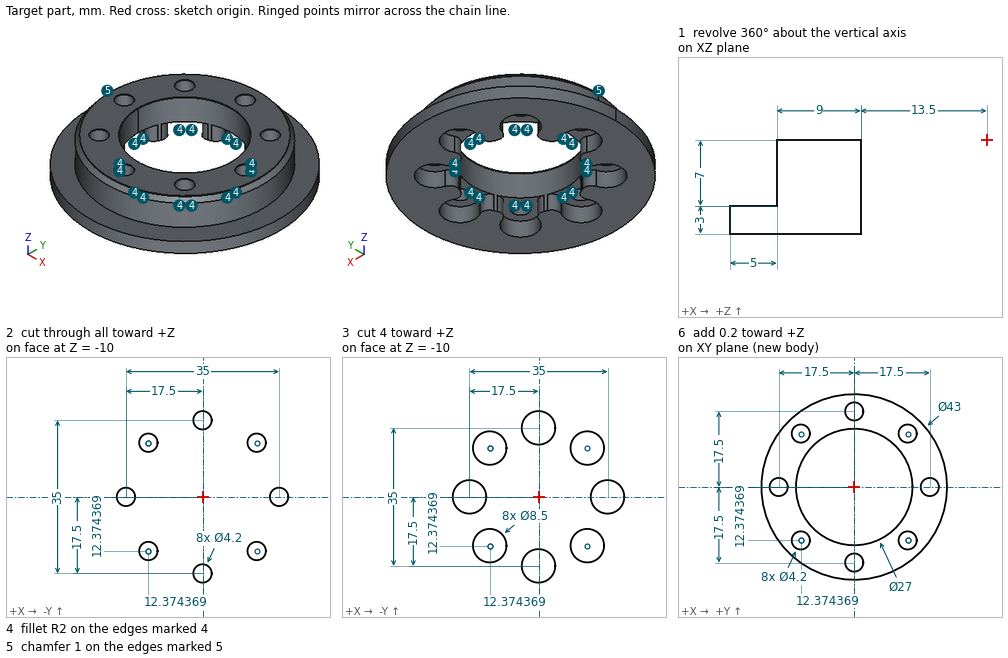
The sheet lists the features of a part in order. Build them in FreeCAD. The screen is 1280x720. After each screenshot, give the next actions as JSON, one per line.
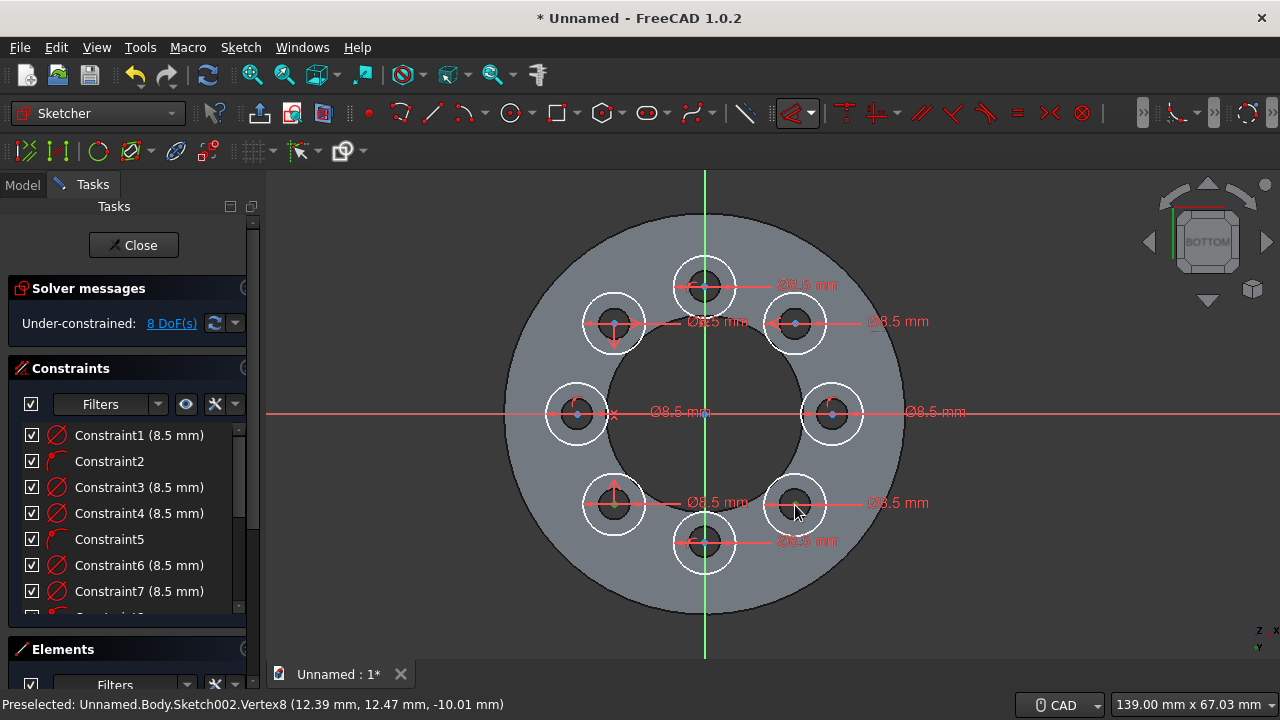
{"action": "left_click", "coordinate": [705, 476]}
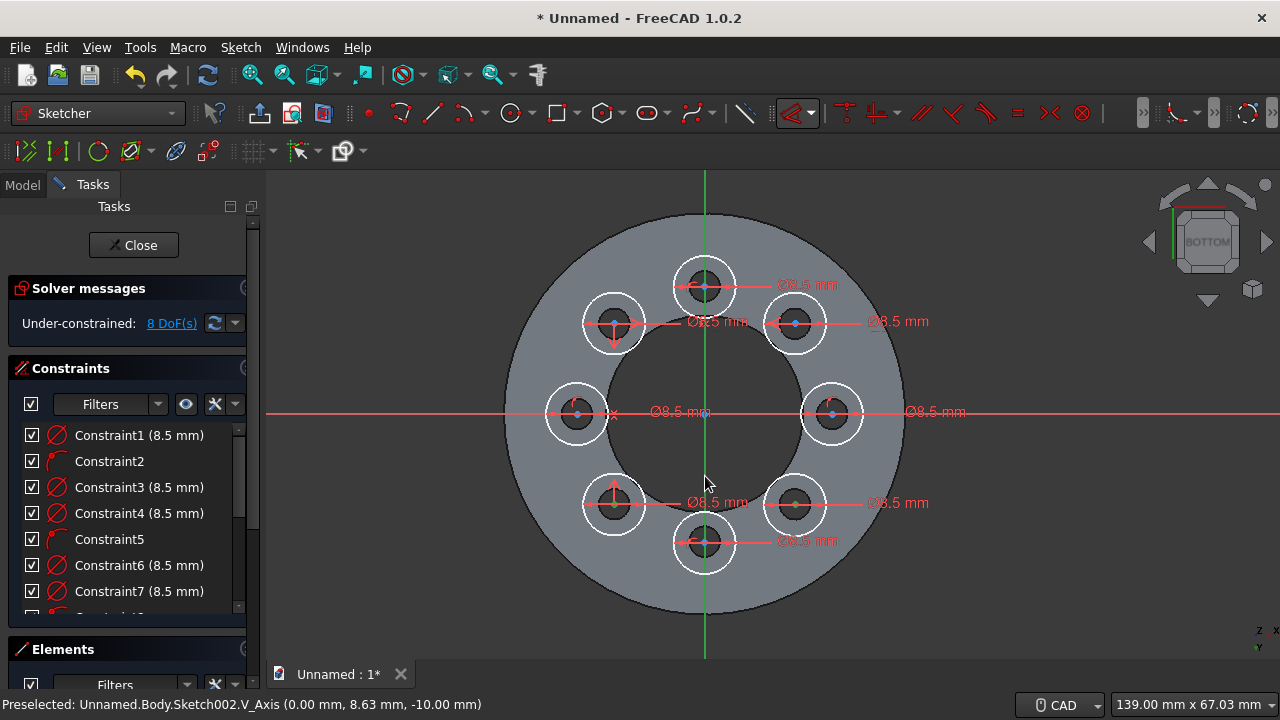
{"action": "key", "text": "s"}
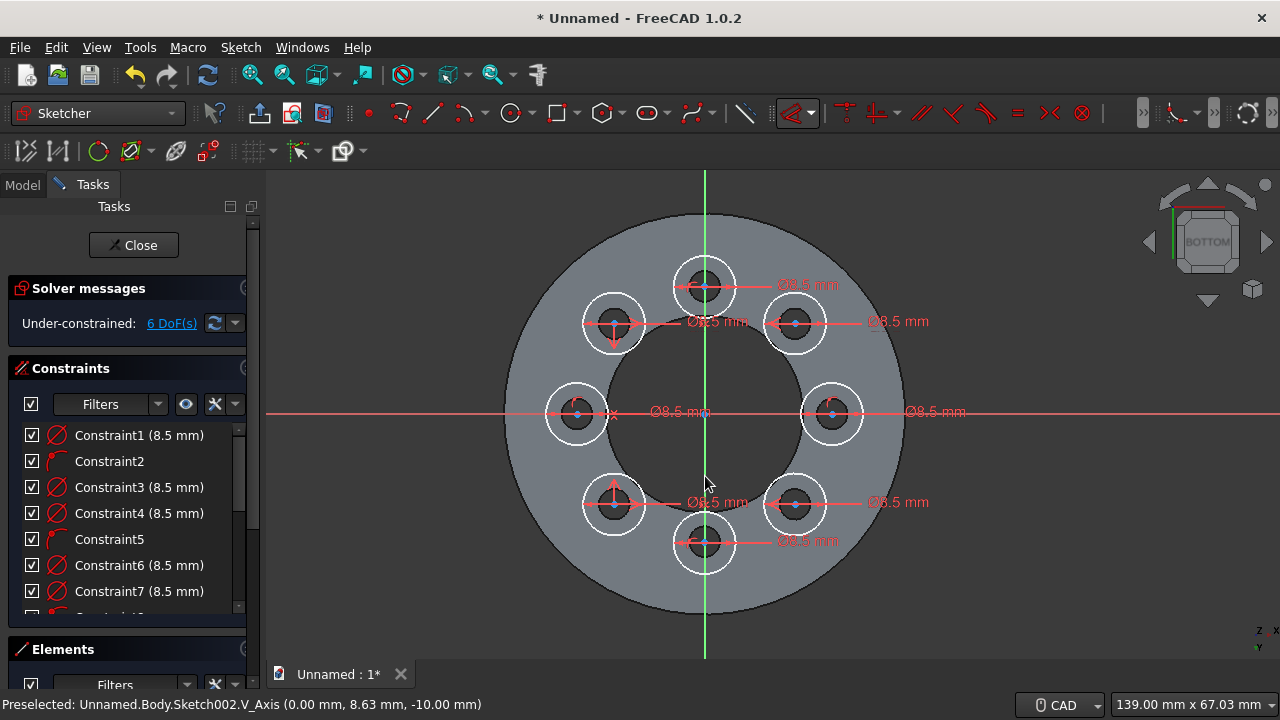
{"action": "left_click", "coordinate": [705, 543]}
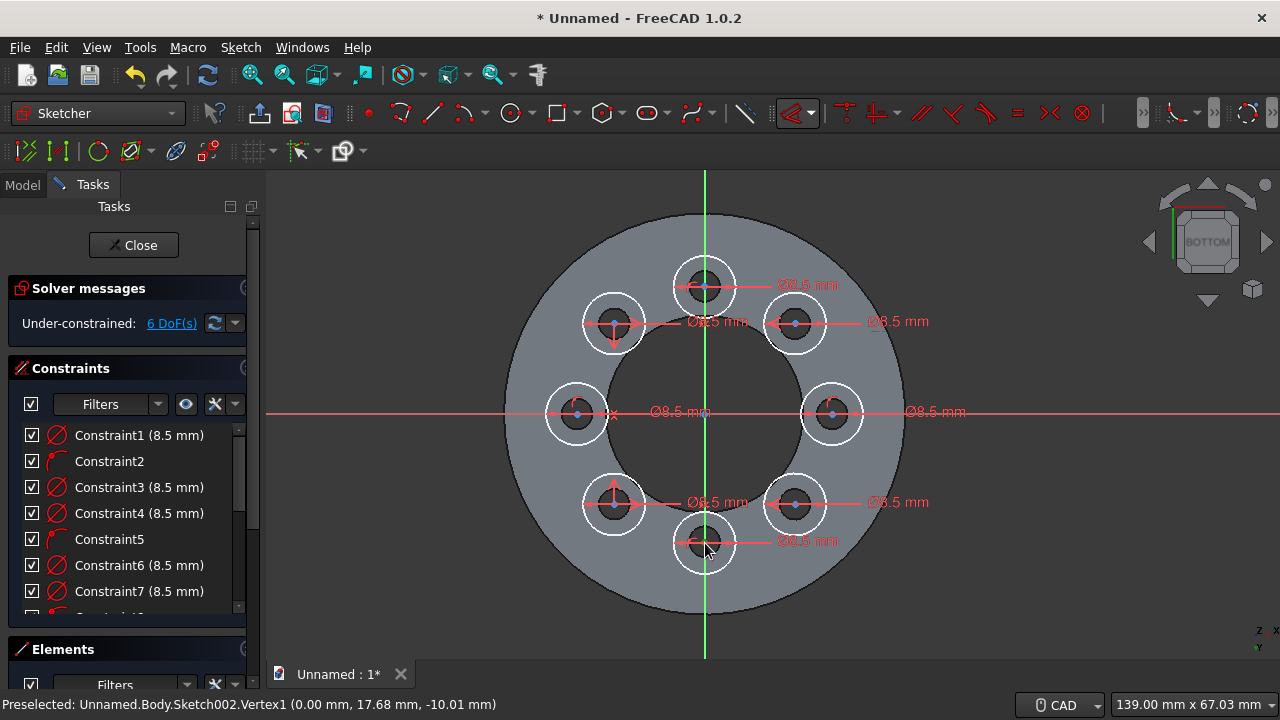
{"action": "left_click", "coordinate": [705, 287]}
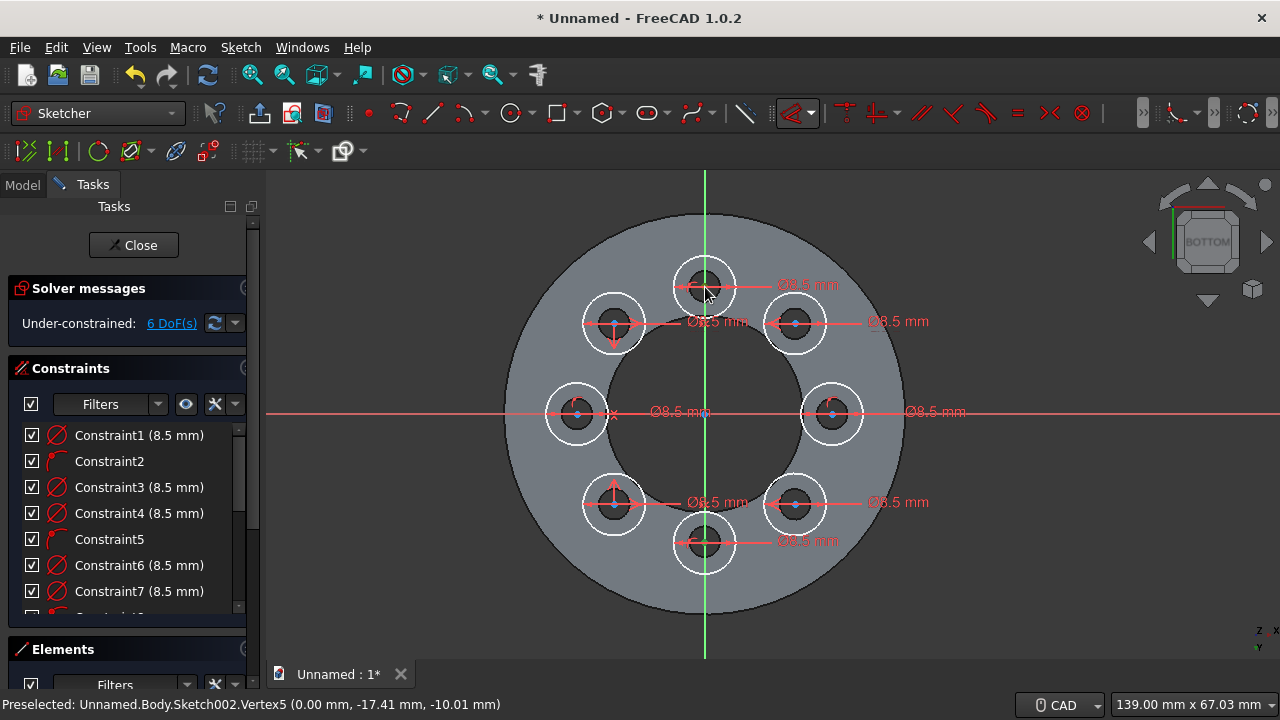
{"action": "key", "text": "i"}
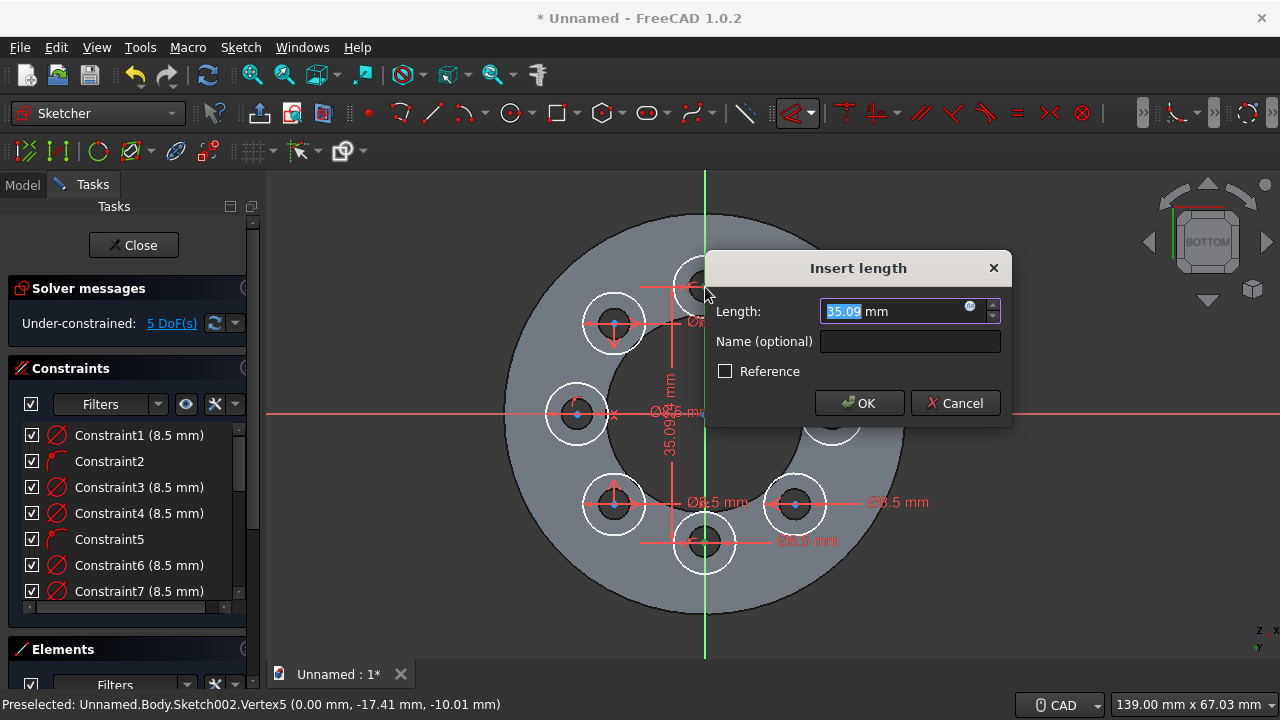
{"action": "type", "text": "35"}
{"action": "key", "text": "Return"}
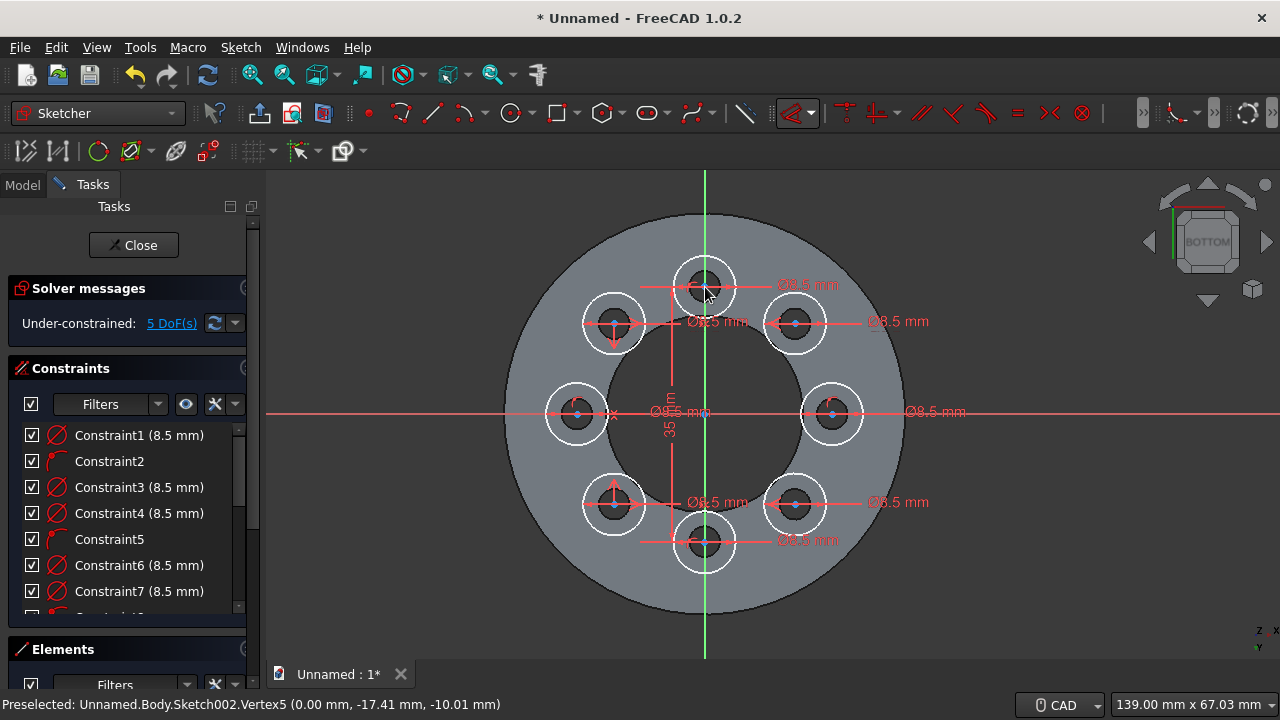
{"action": "left_click", "coordinate": [577, 414]}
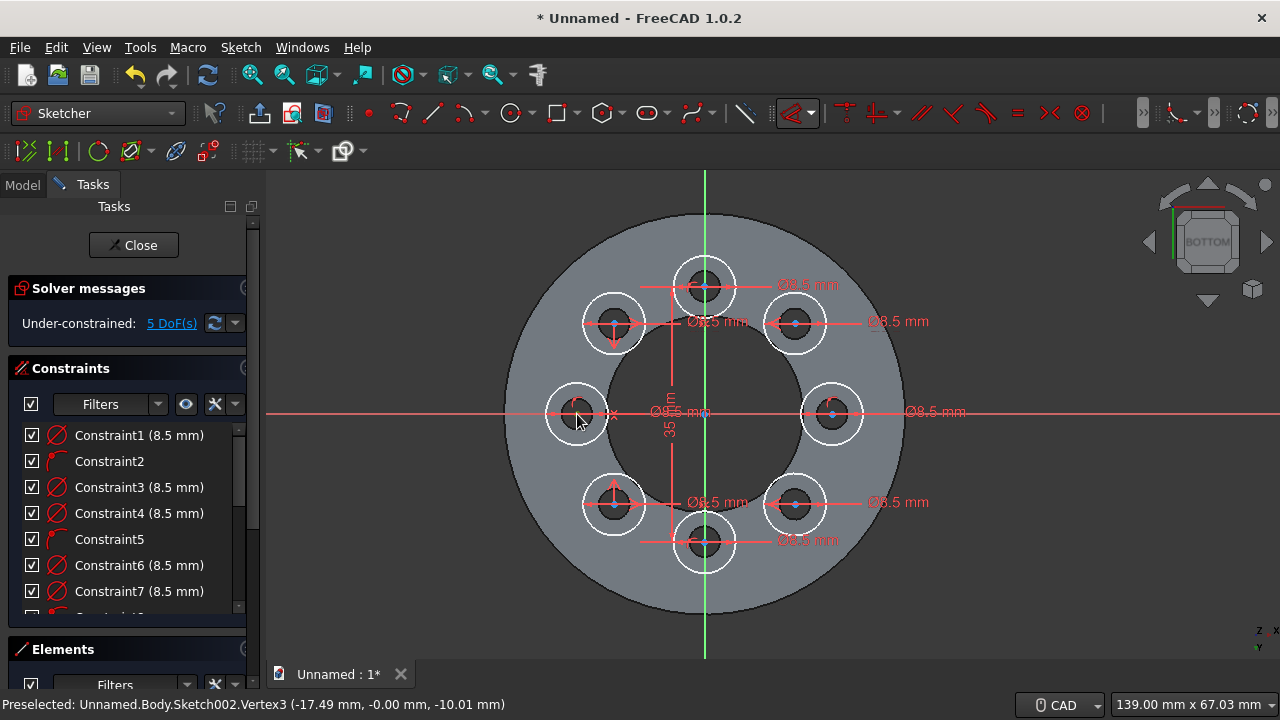
{"action": "left_click", "coordinate": [832, 414]}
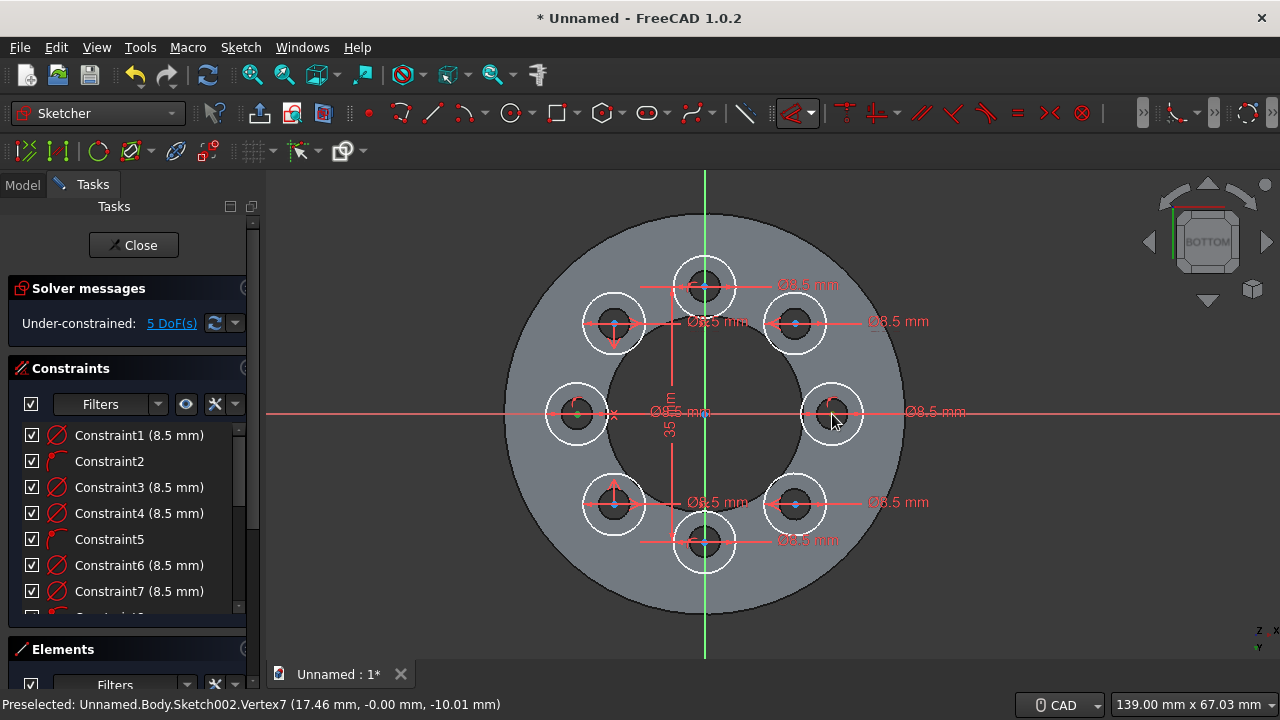
{"action": "left_click", "coordinate": [814, 114]}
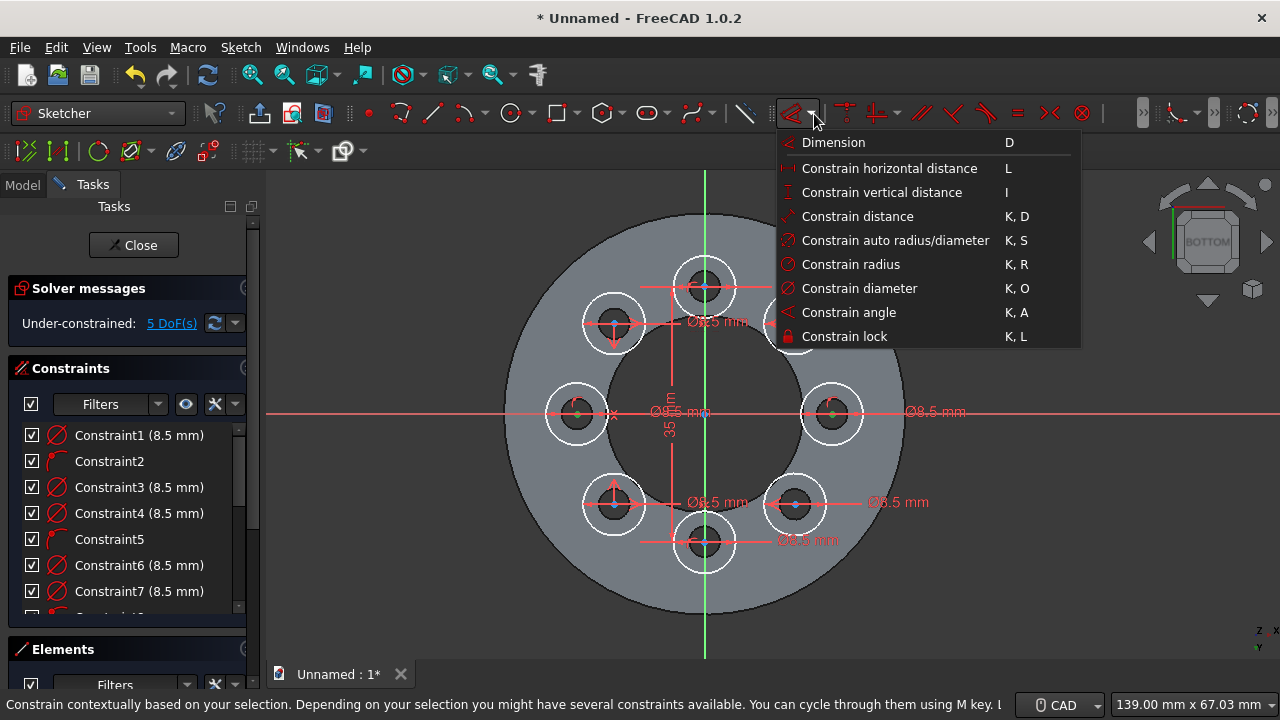
{"action": "left_click", "coordinate": [929, 168]}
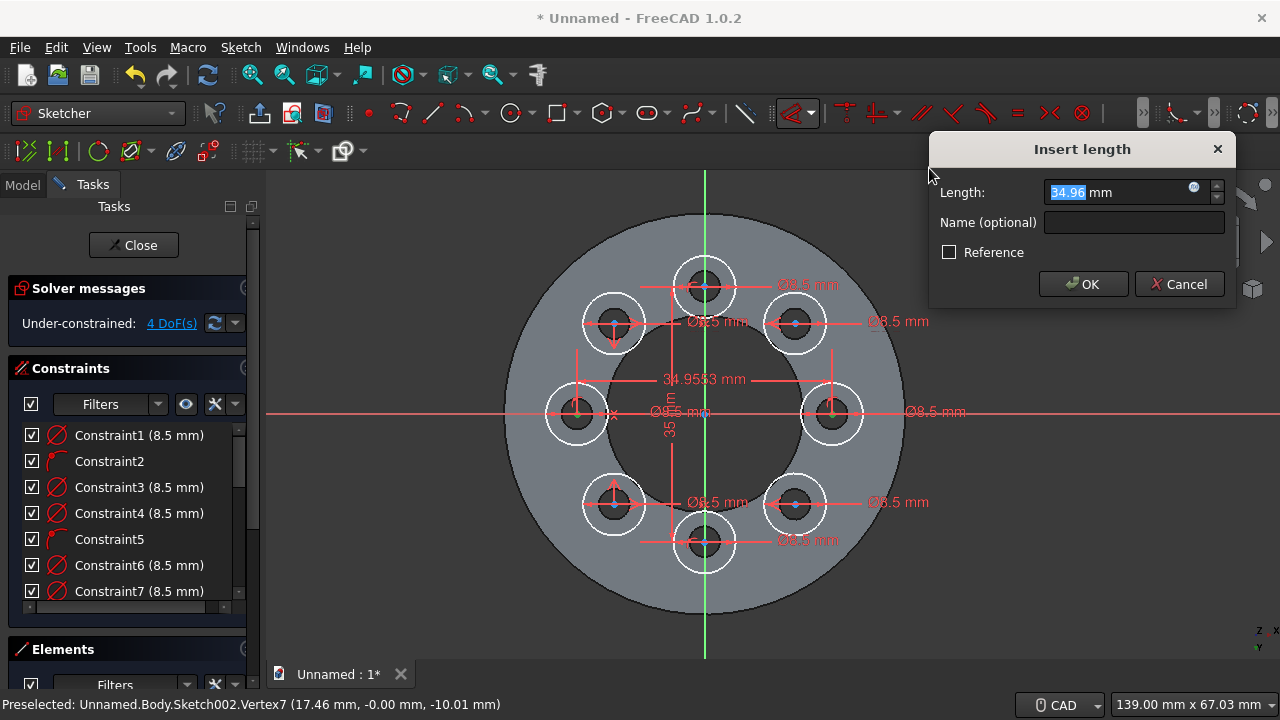
{"action": "type", "text": "35"}
{"action": "key", "text": "Return"}